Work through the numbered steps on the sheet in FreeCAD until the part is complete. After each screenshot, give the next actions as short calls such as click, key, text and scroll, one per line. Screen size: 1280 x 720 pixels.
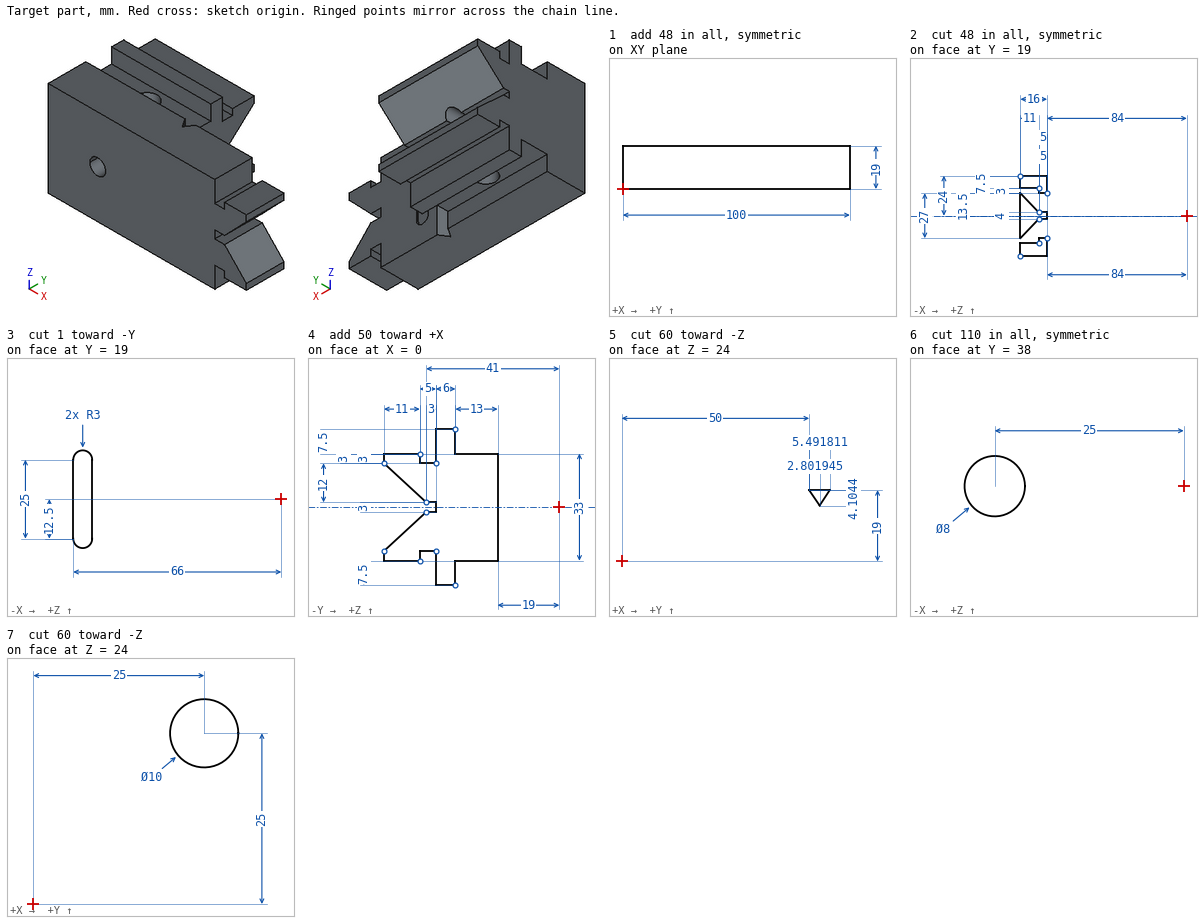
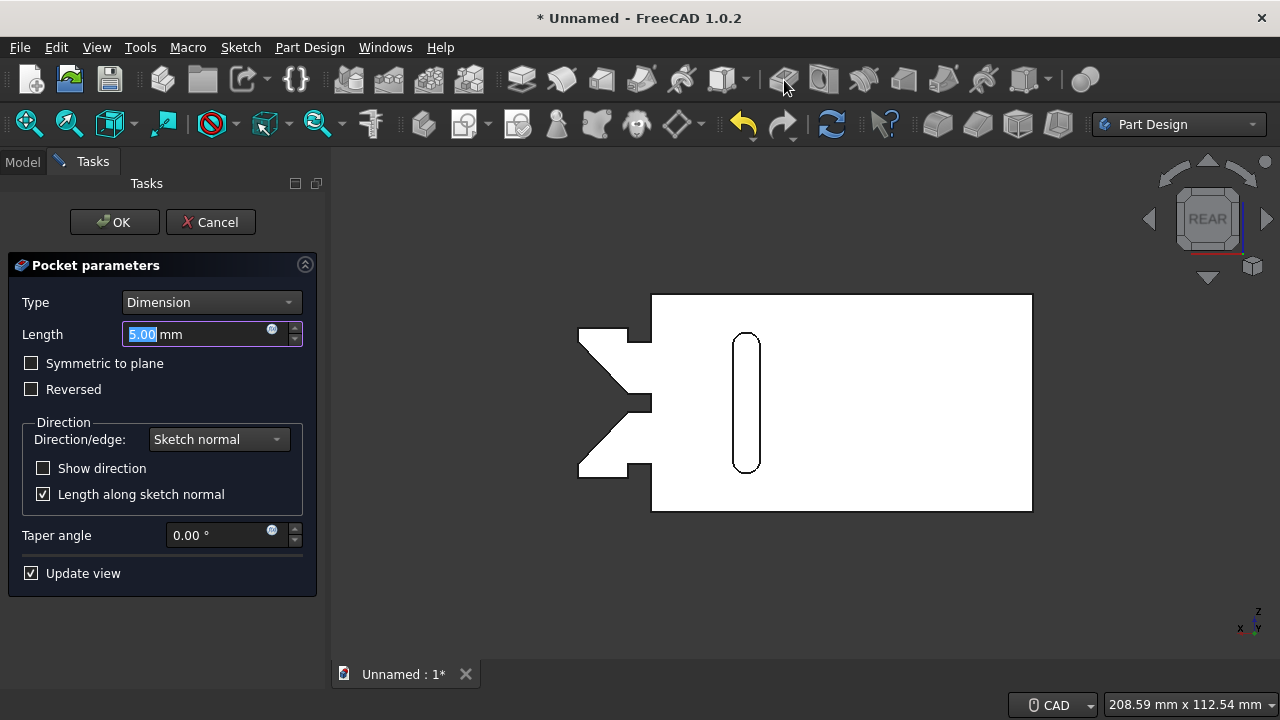
text(1)
key(Tab)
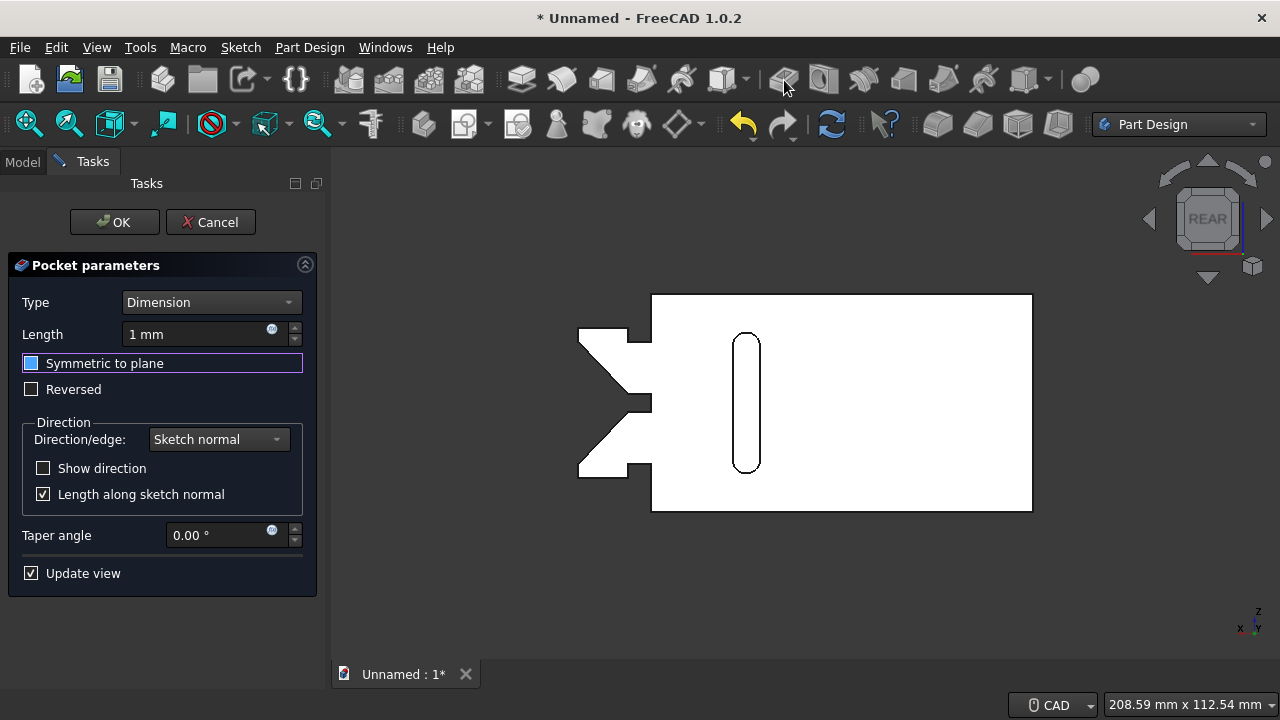
click(115, 222)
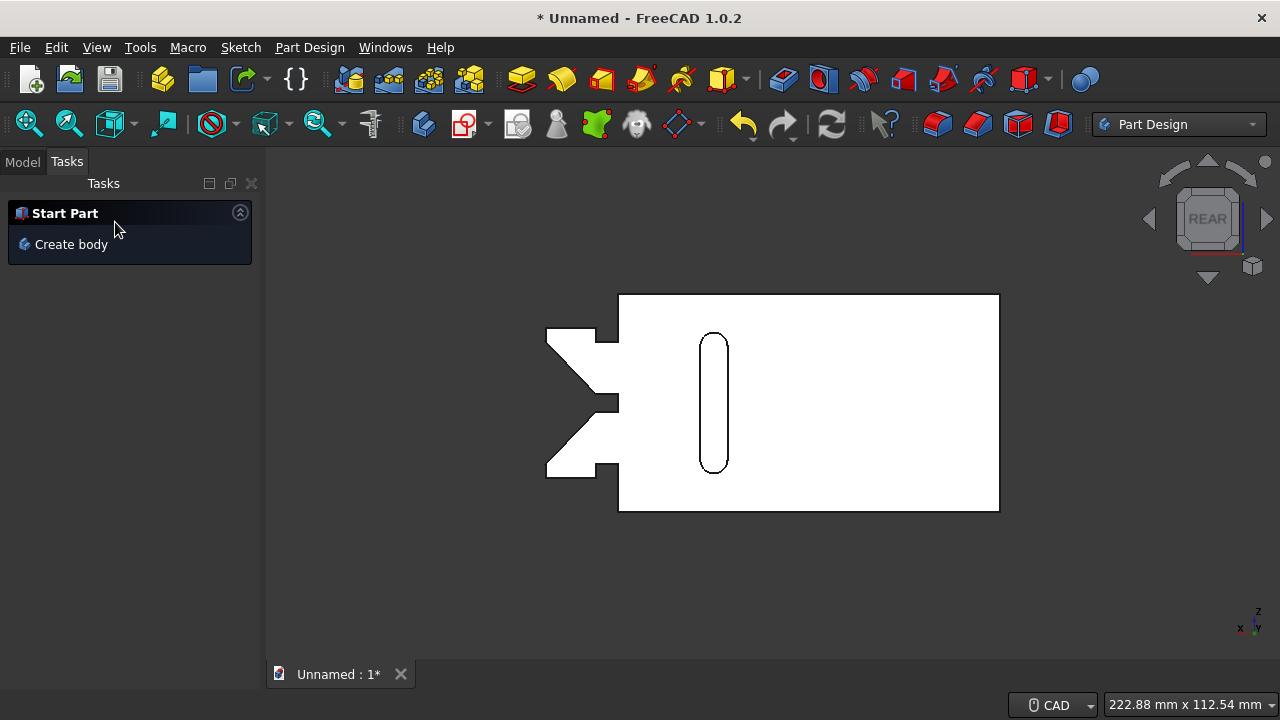
click(30, 124)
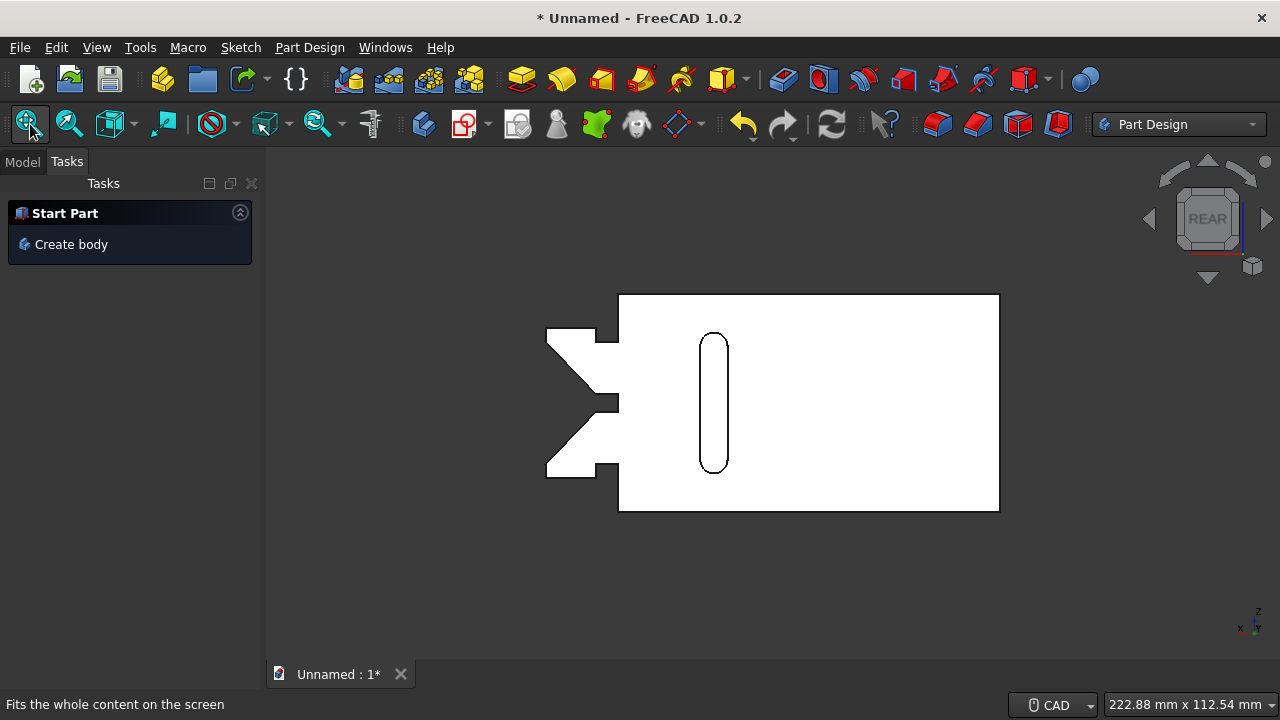
key(6)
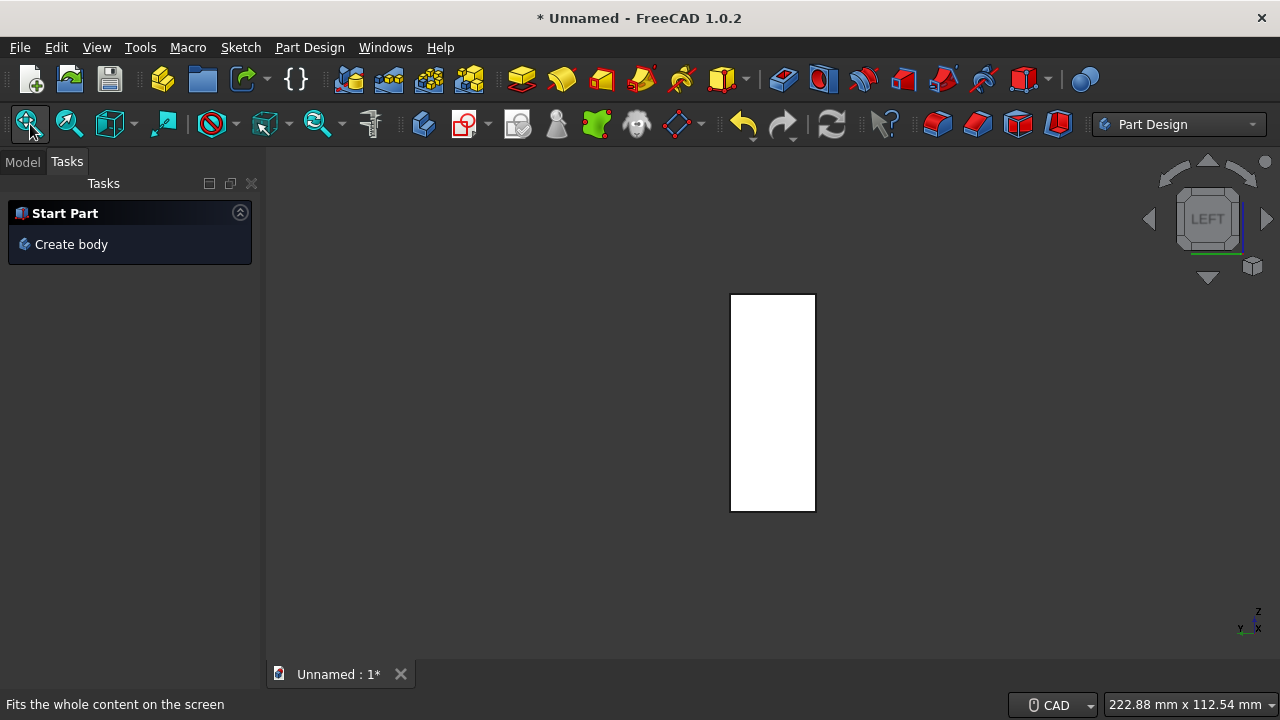
click(30, 124)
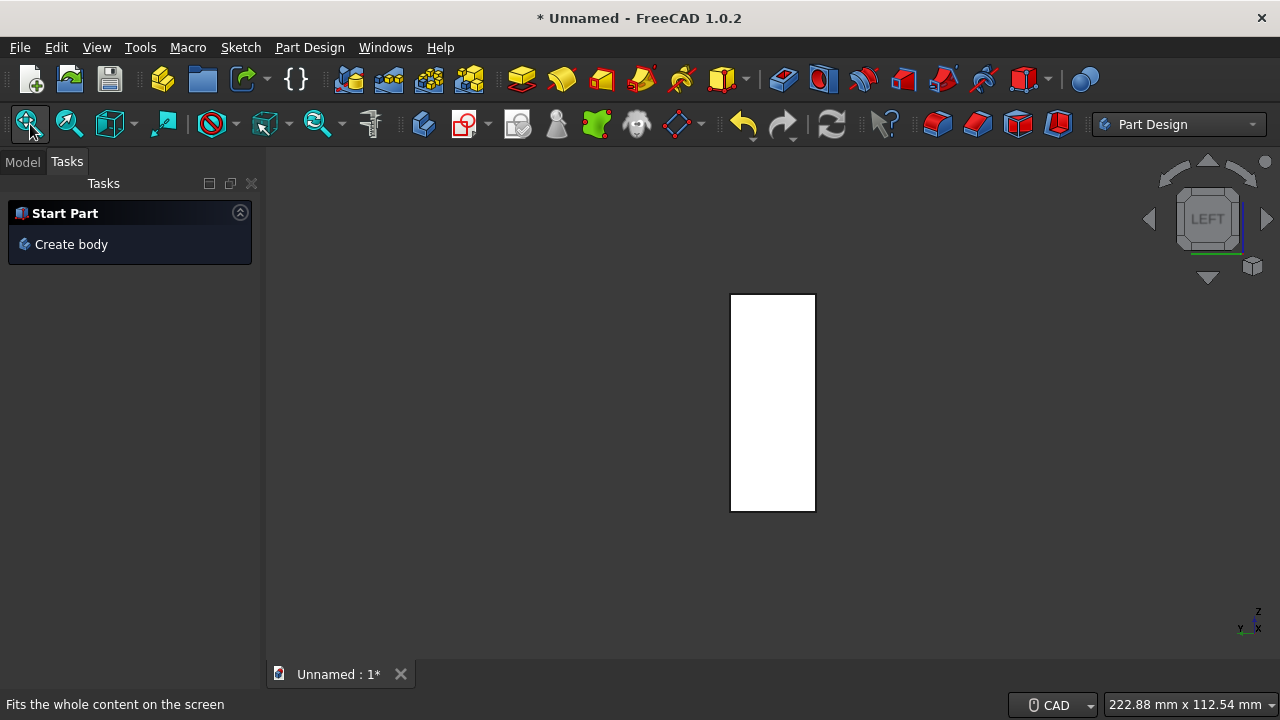
click(773, 340)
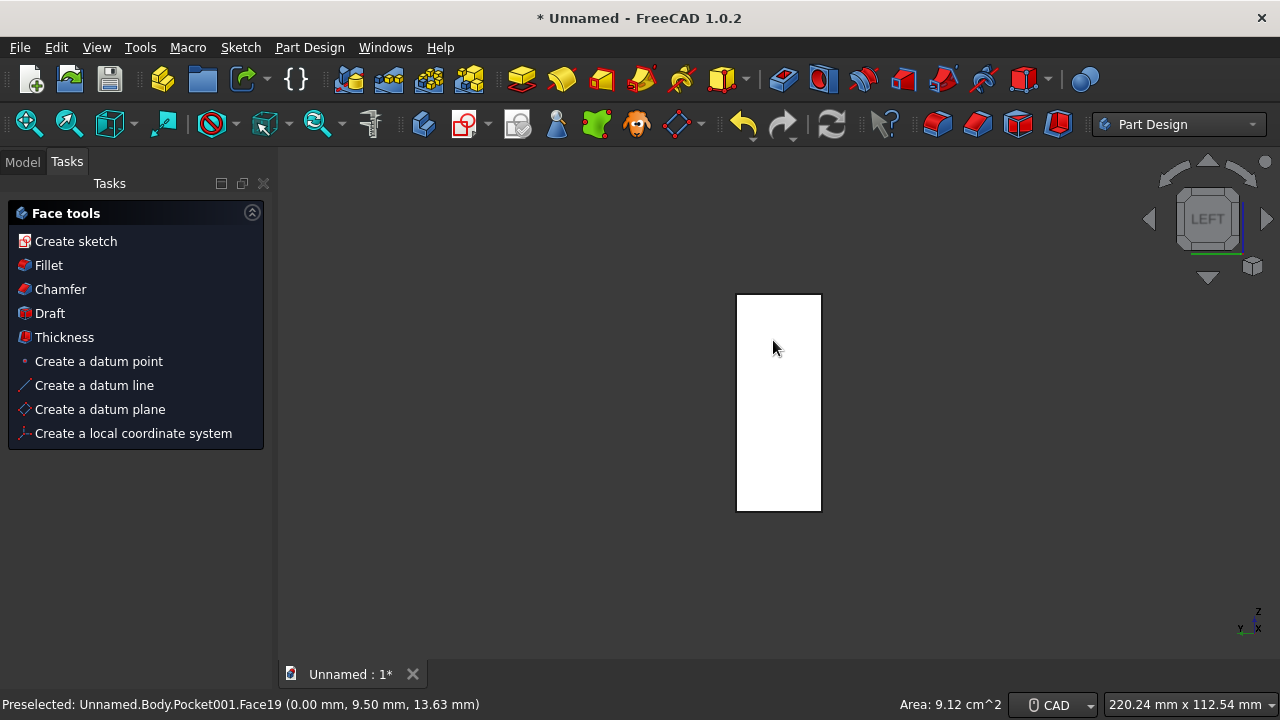
click(464, 124)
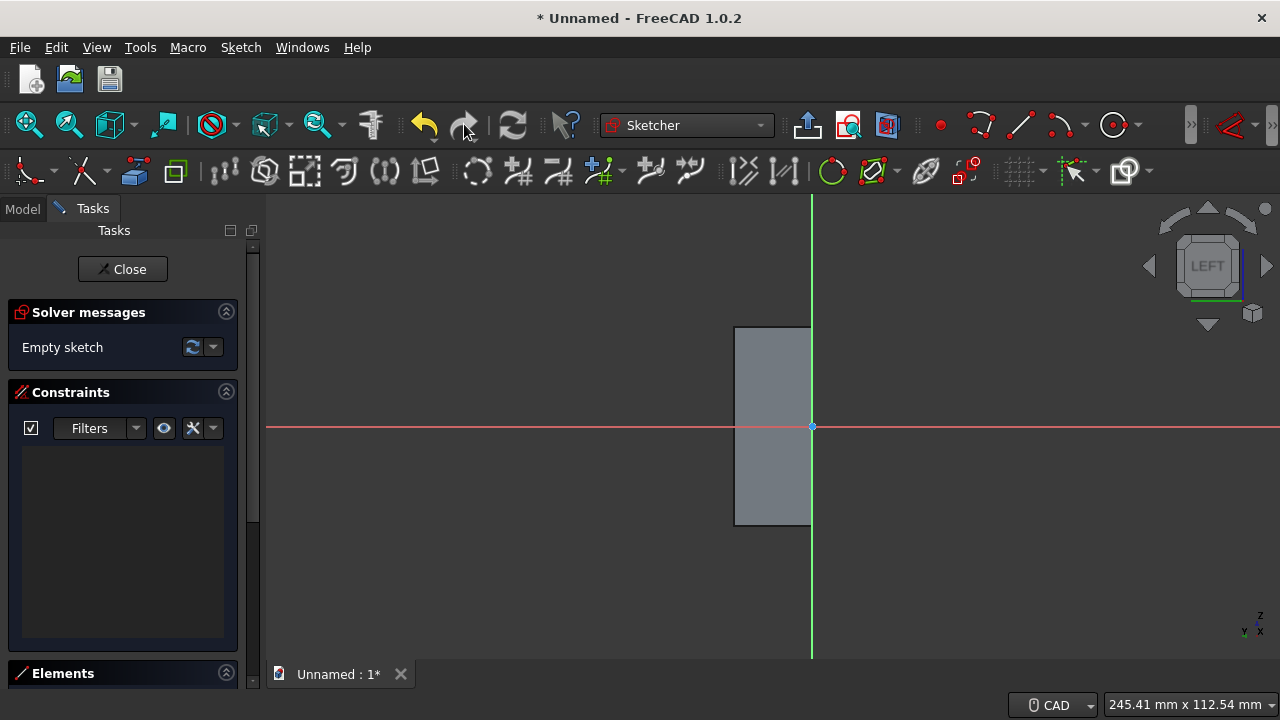
scroll(693, 426, up, 2)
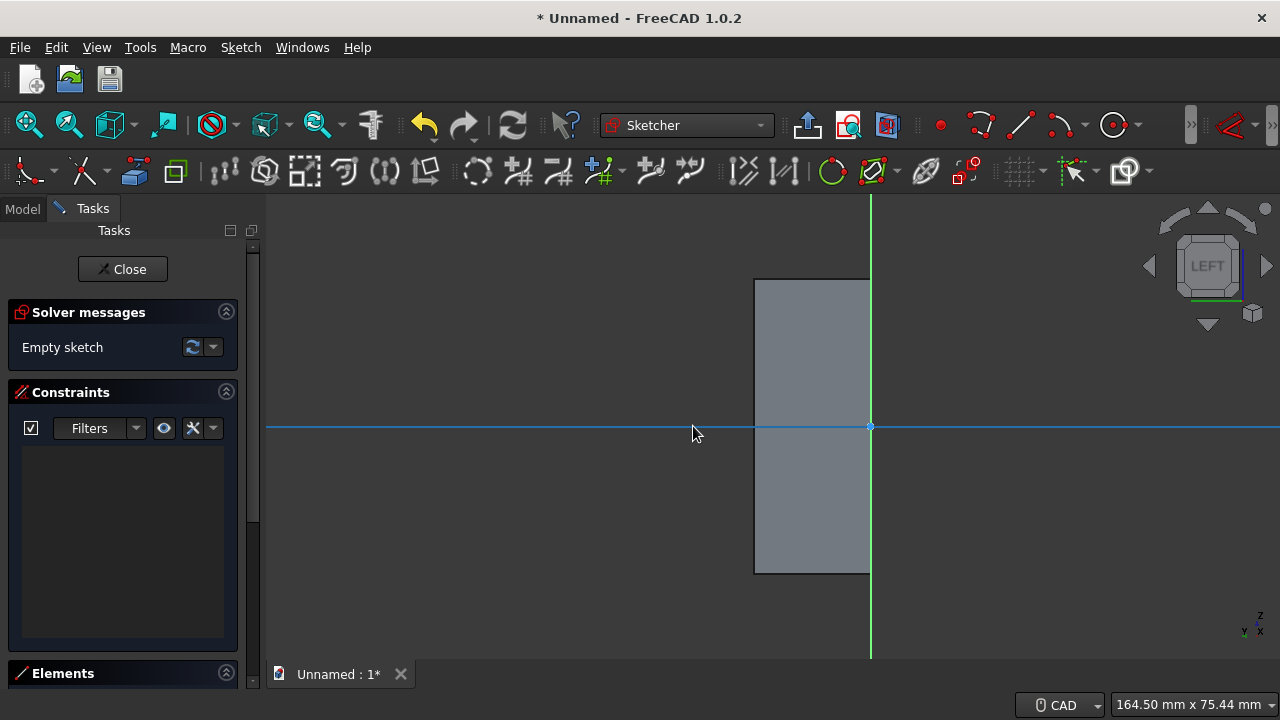
click(982, 126)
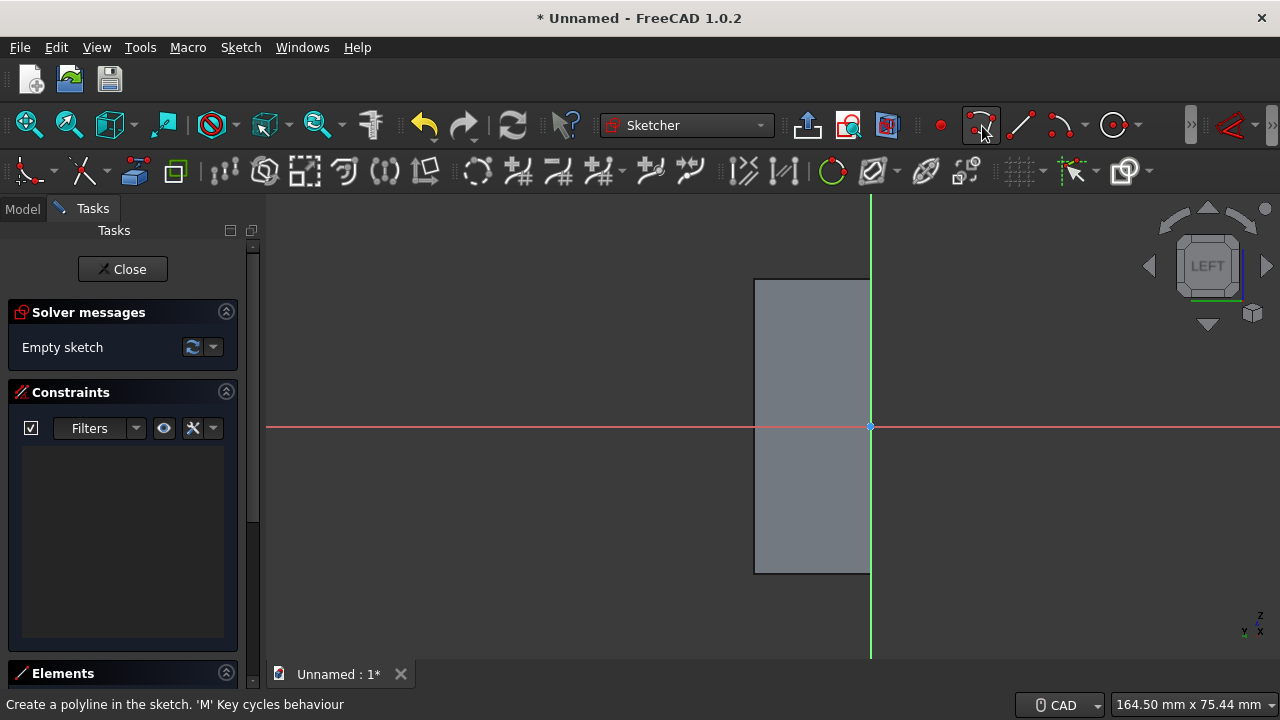
click(754, 528)
click(754, 325)
click(673, 325)
click(673, 279)
click(636, 279)
click(636, 343)
click(606, 343)
click(606, 325)
click(538, 325)
click(538, 343)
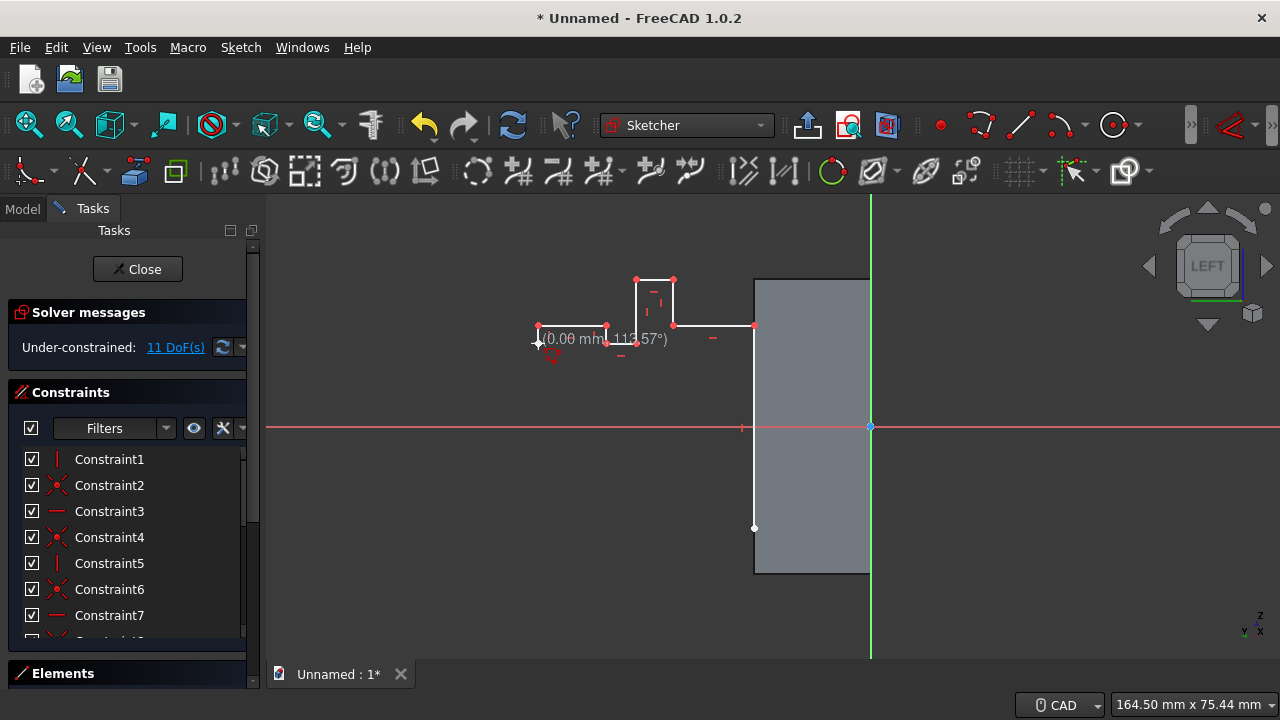
scroll(618, 417, up, 3)